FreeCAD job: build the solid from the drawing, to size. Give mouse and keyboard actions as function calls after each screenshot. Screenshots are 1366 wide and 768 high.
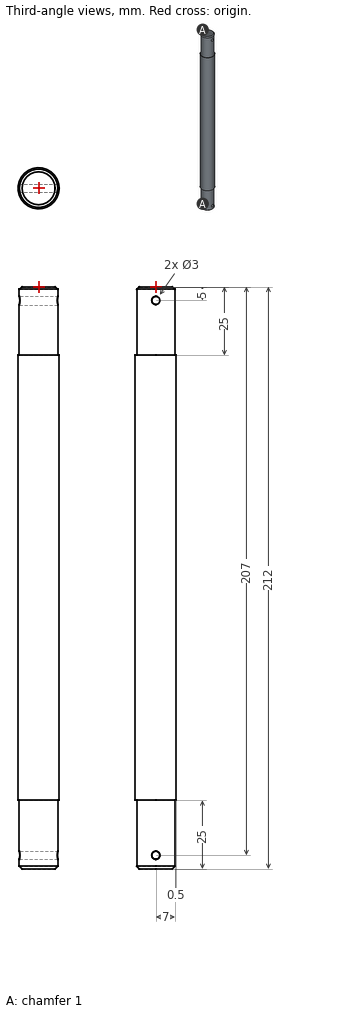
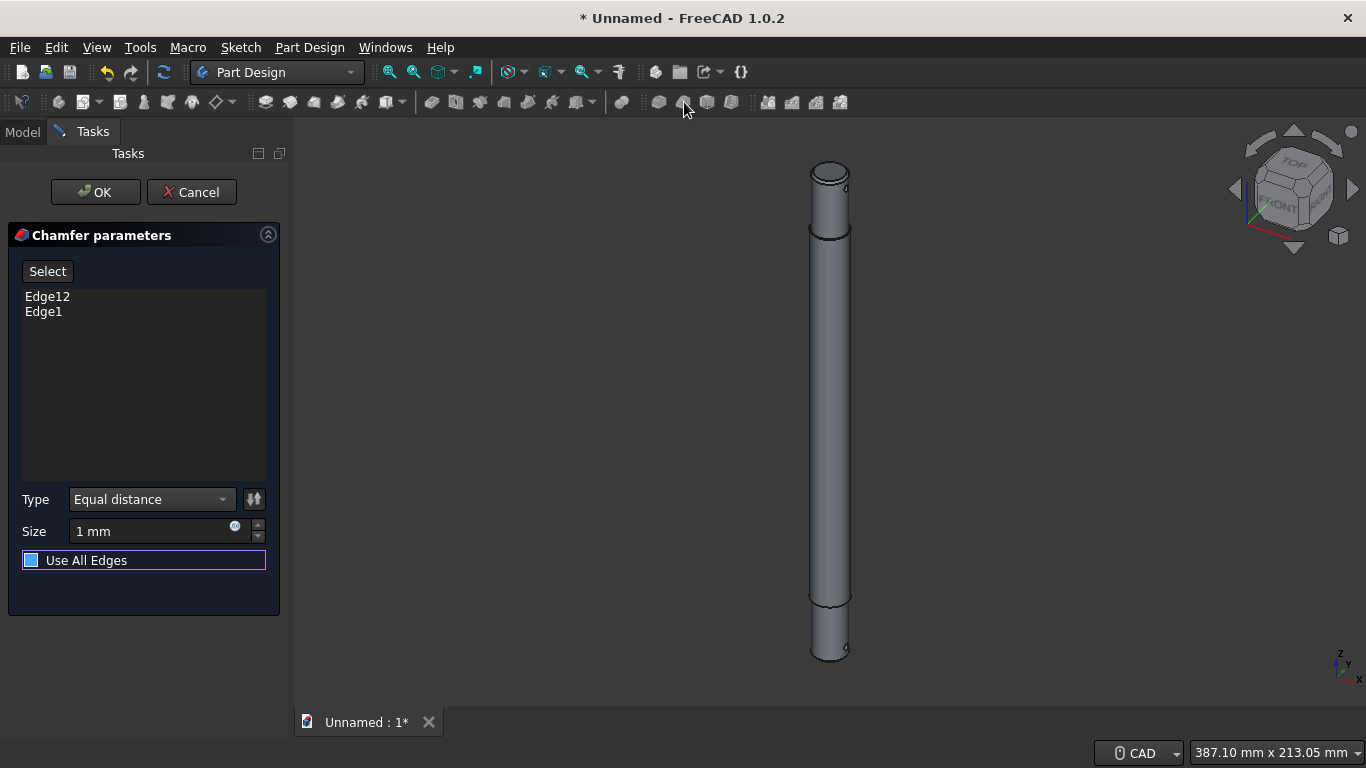
click(96, 192)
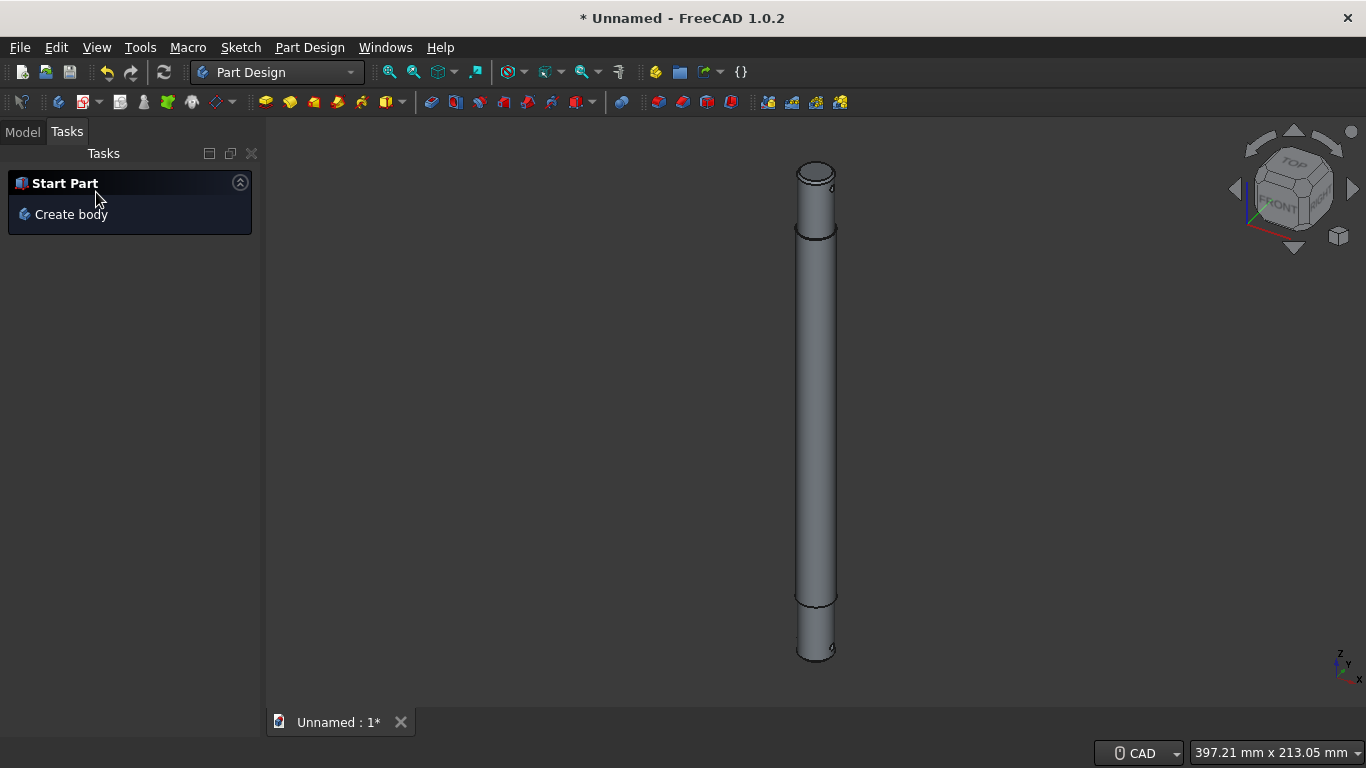
key(0)